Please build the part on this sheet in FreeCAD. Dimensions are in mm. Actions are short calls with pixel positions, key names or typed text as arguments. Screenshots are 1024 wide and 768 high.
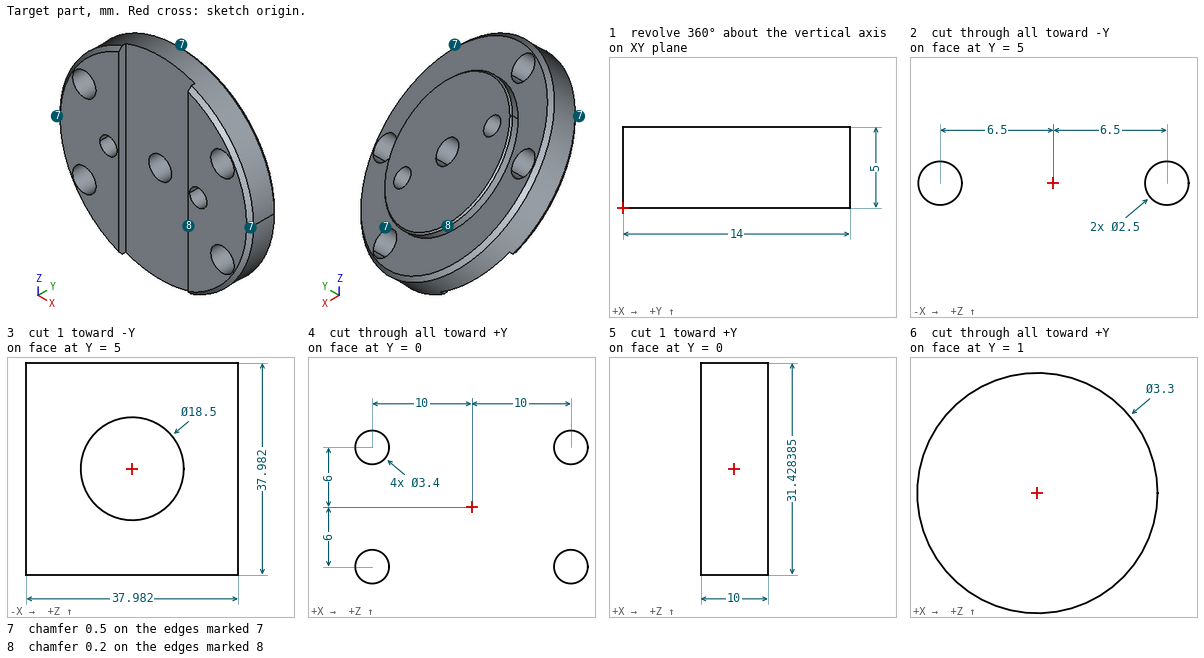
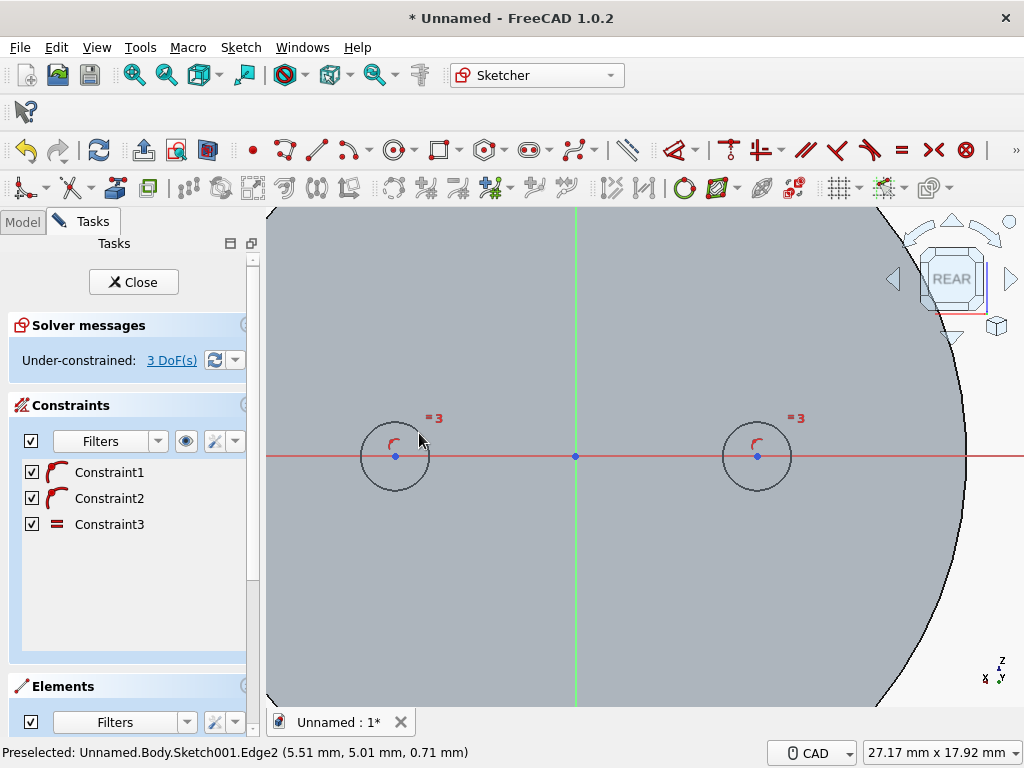
key(d)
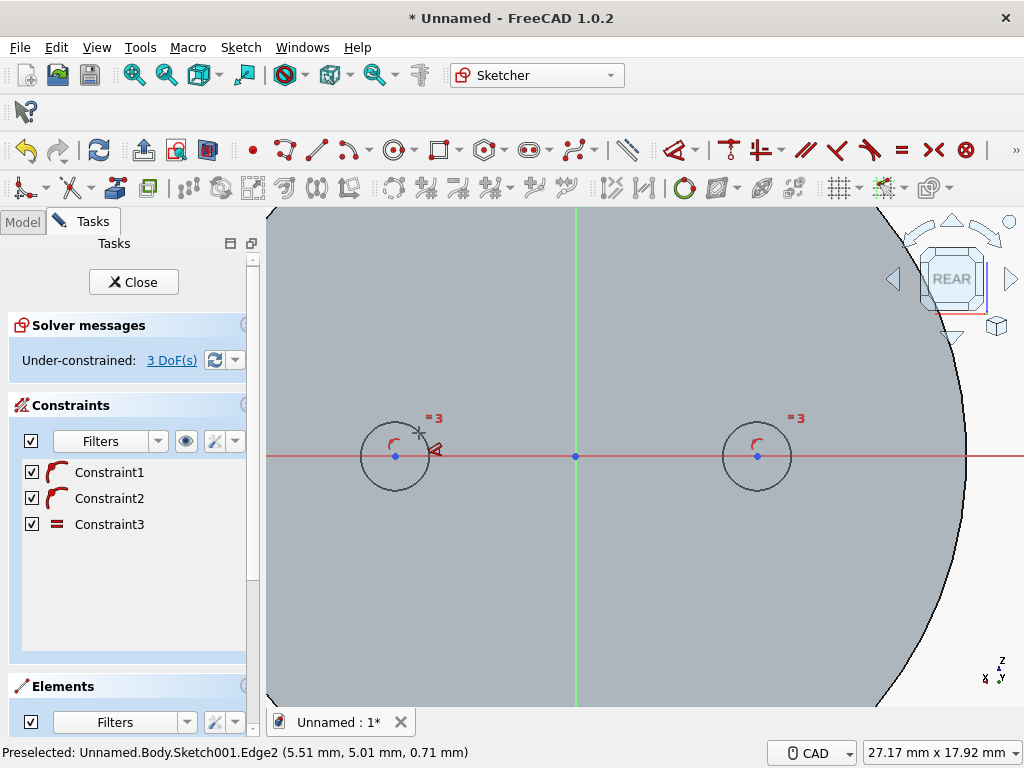
click(781, 432)
click(803, 409)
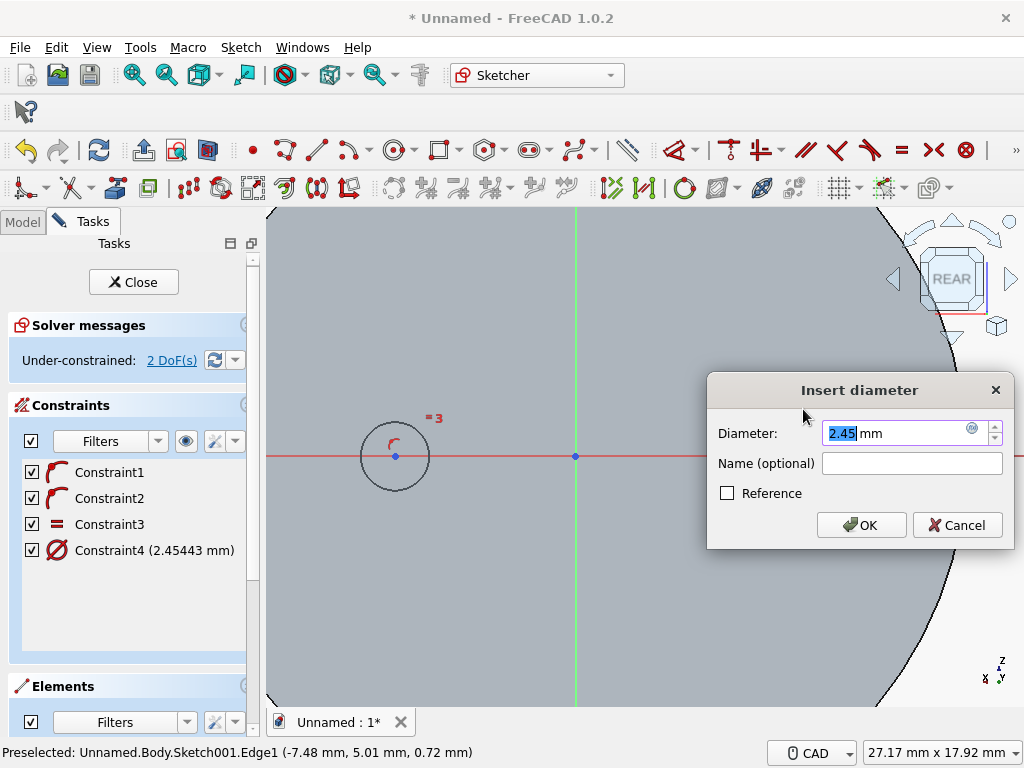
text(2.5)
key(Return)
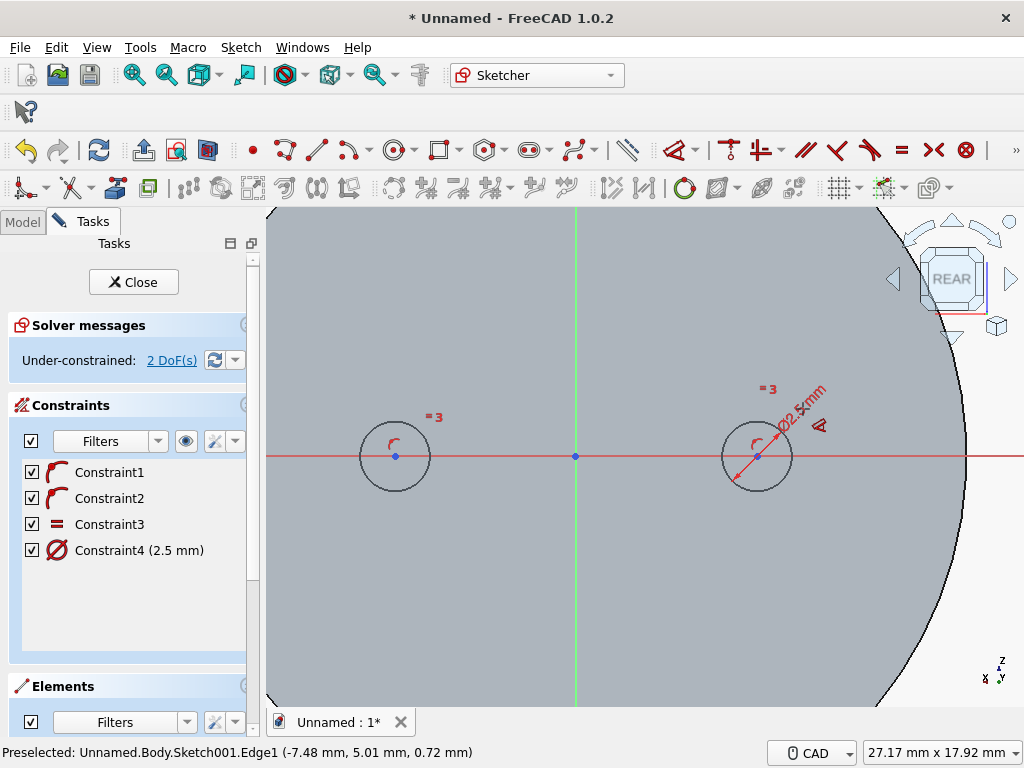
click(757, 456)
click(666, 490)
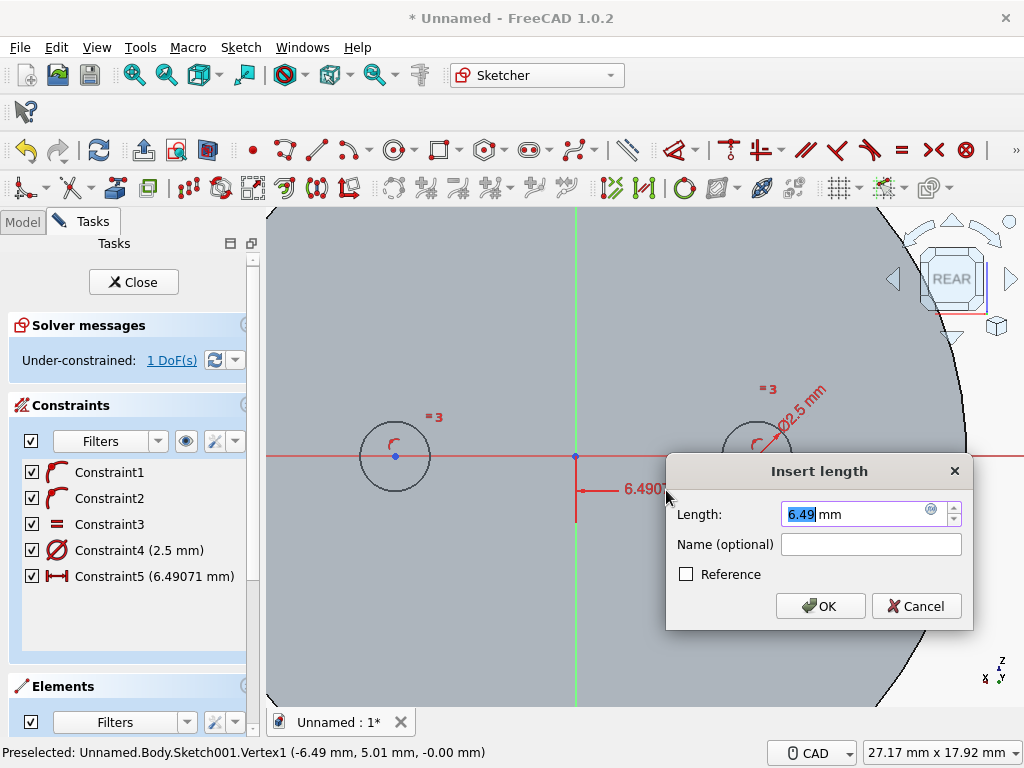
text(6.5)
key(Return)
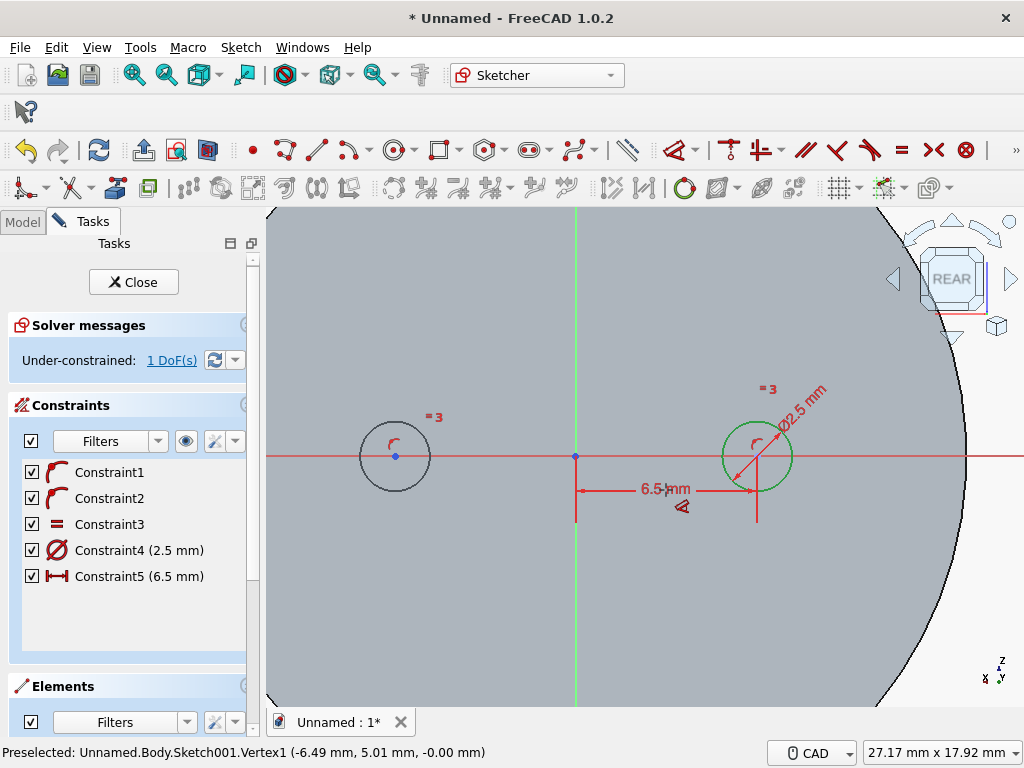
click(395, 456)
click(485, 490)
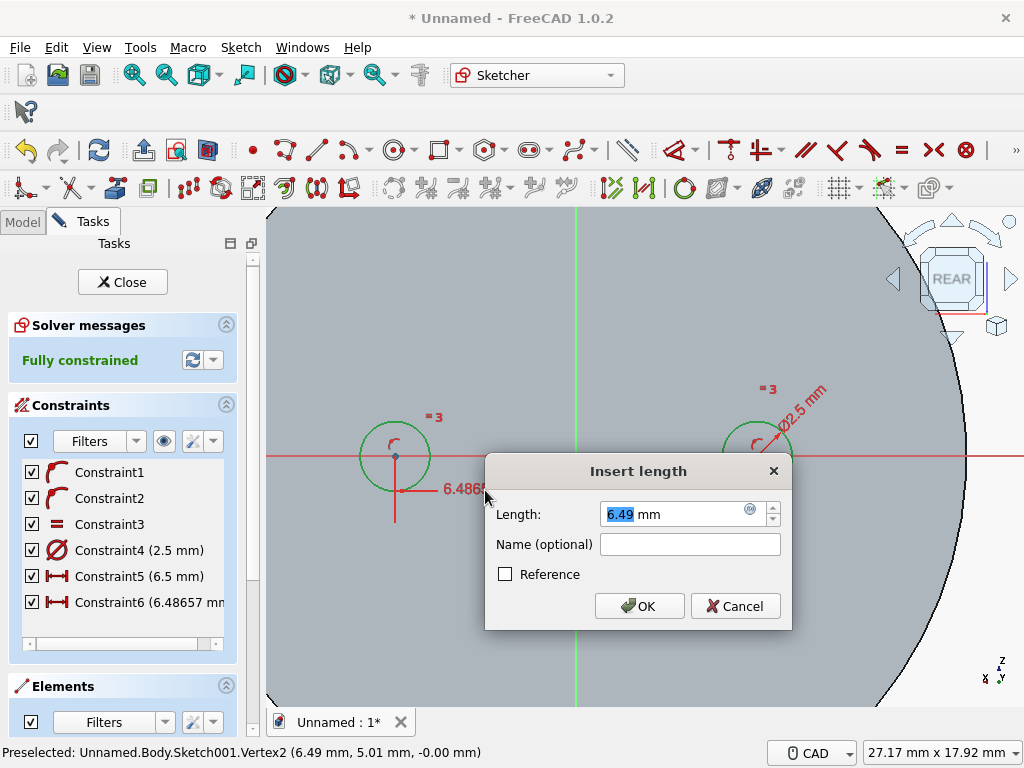
text(6.5)
key(Return)
key(Escape)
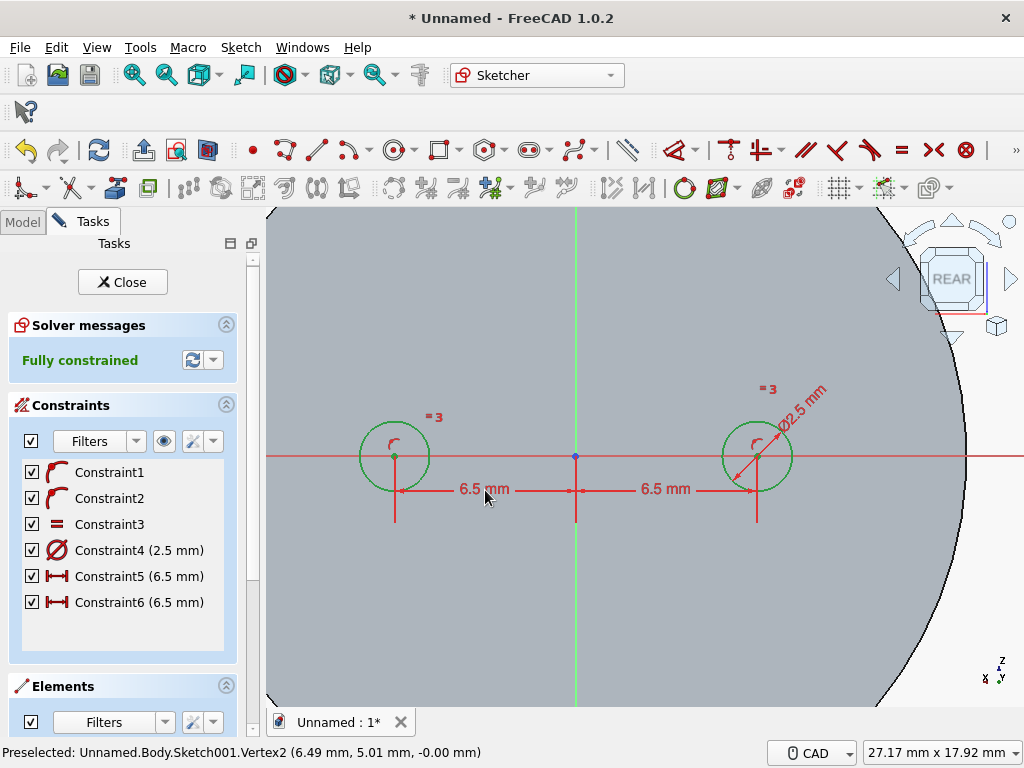
click(123, 282)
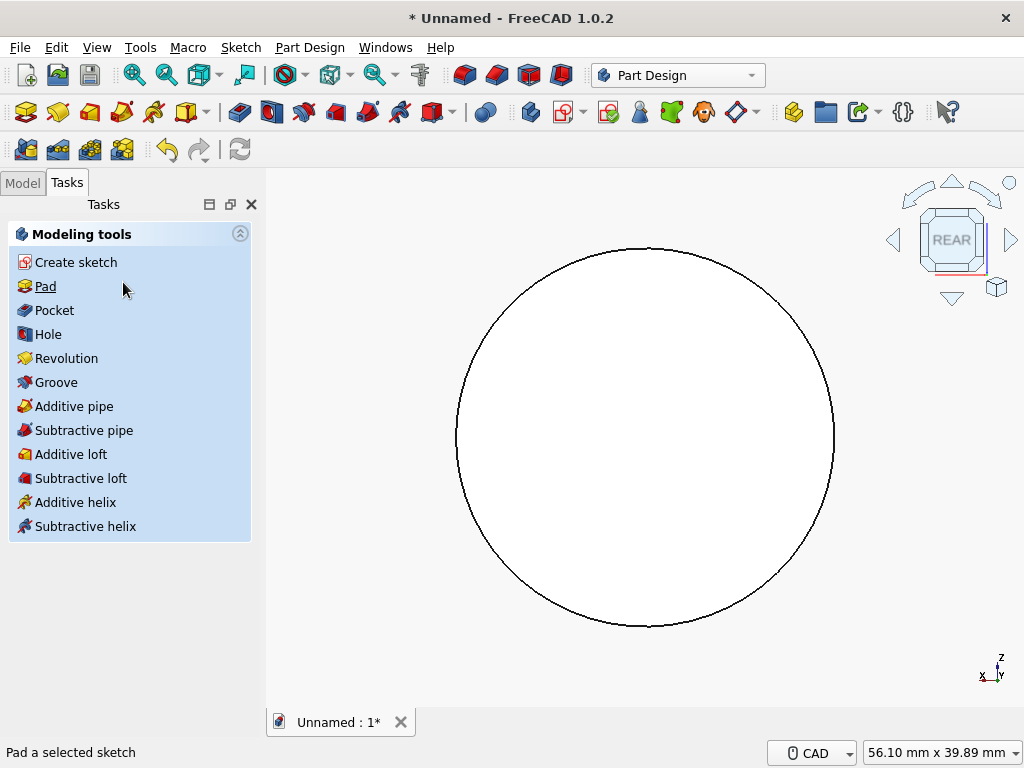
click(240, 112)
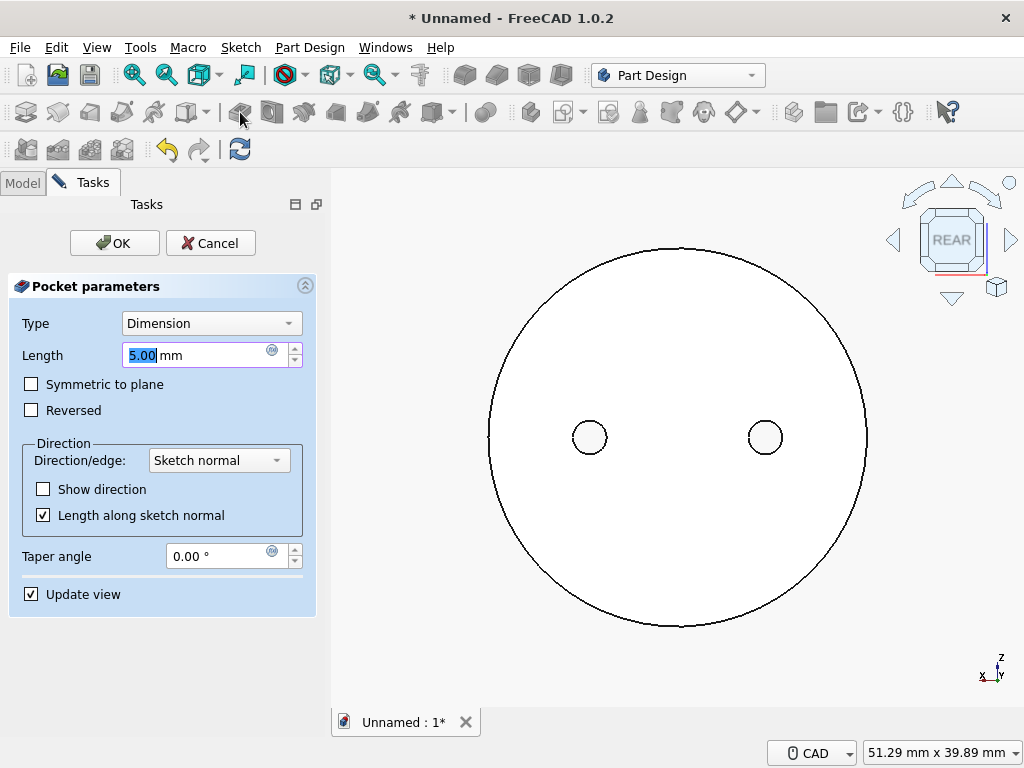
click(212, 324)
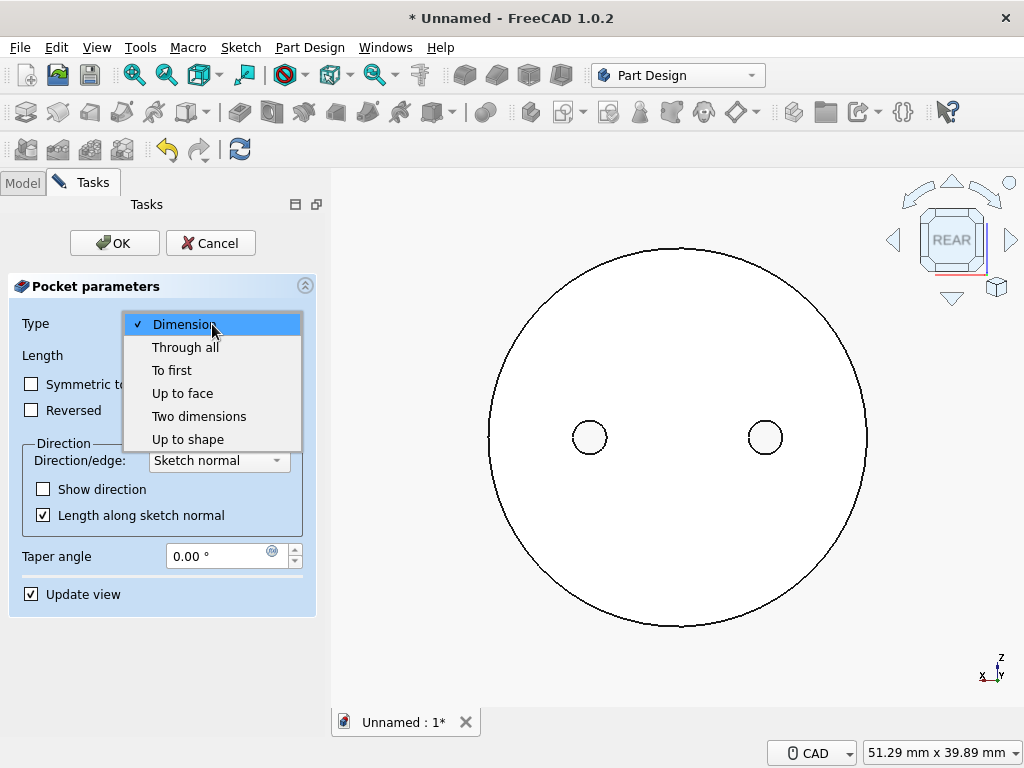
click(212, 348)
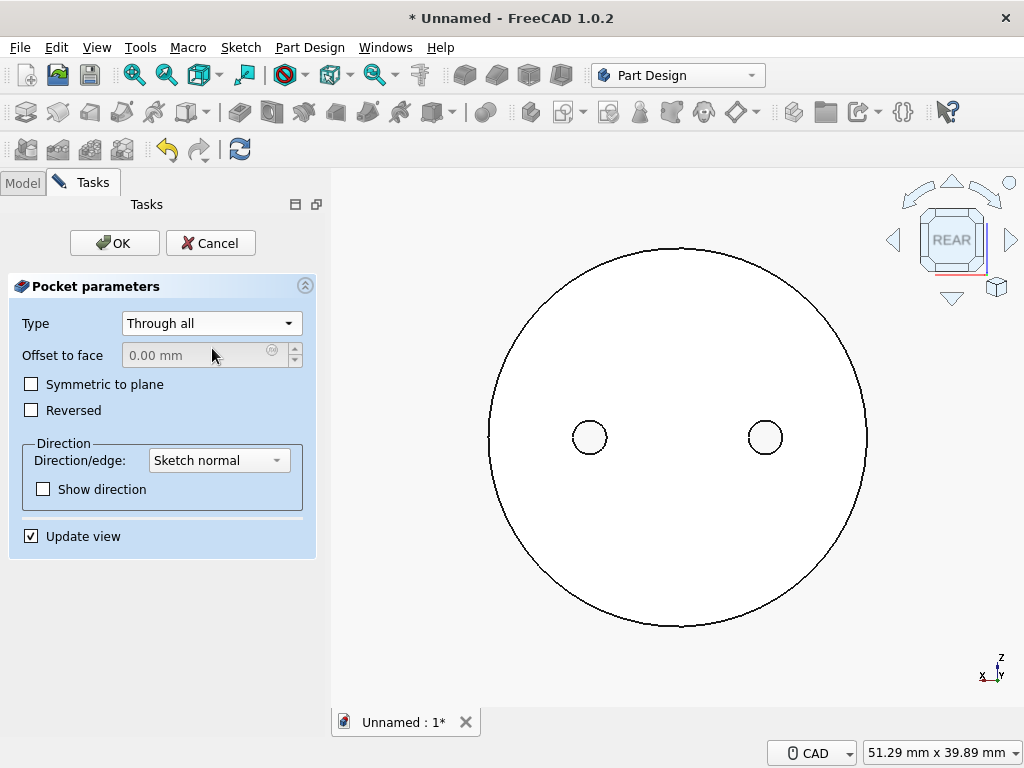
click(115, 243)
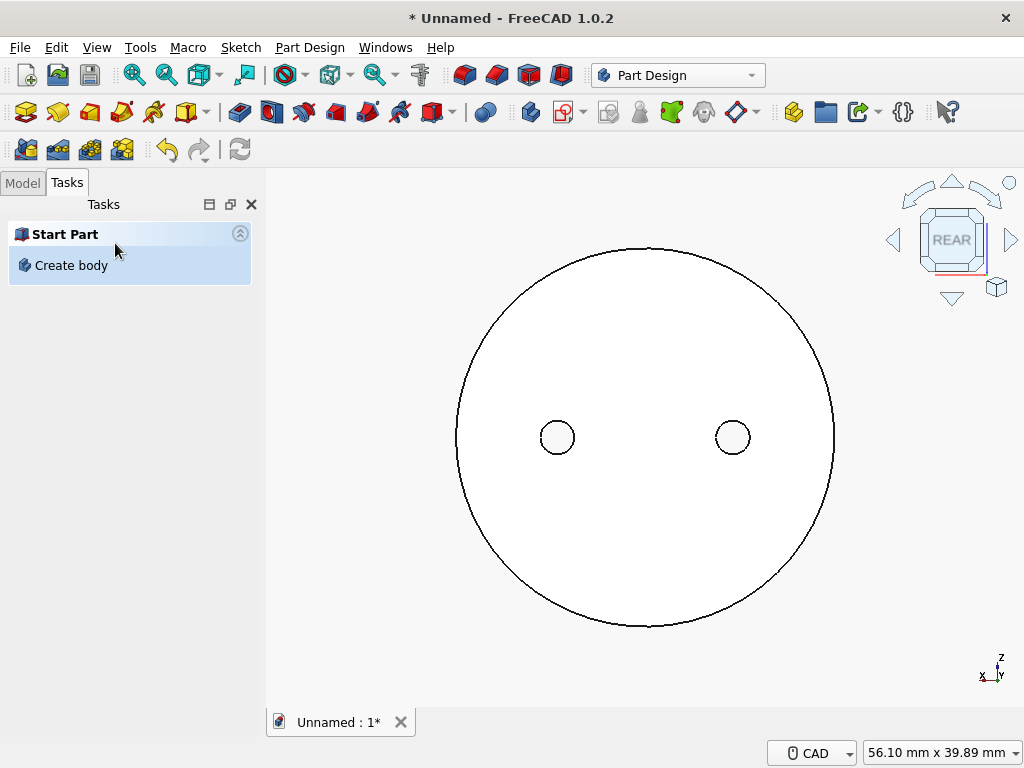
click(645, 382)